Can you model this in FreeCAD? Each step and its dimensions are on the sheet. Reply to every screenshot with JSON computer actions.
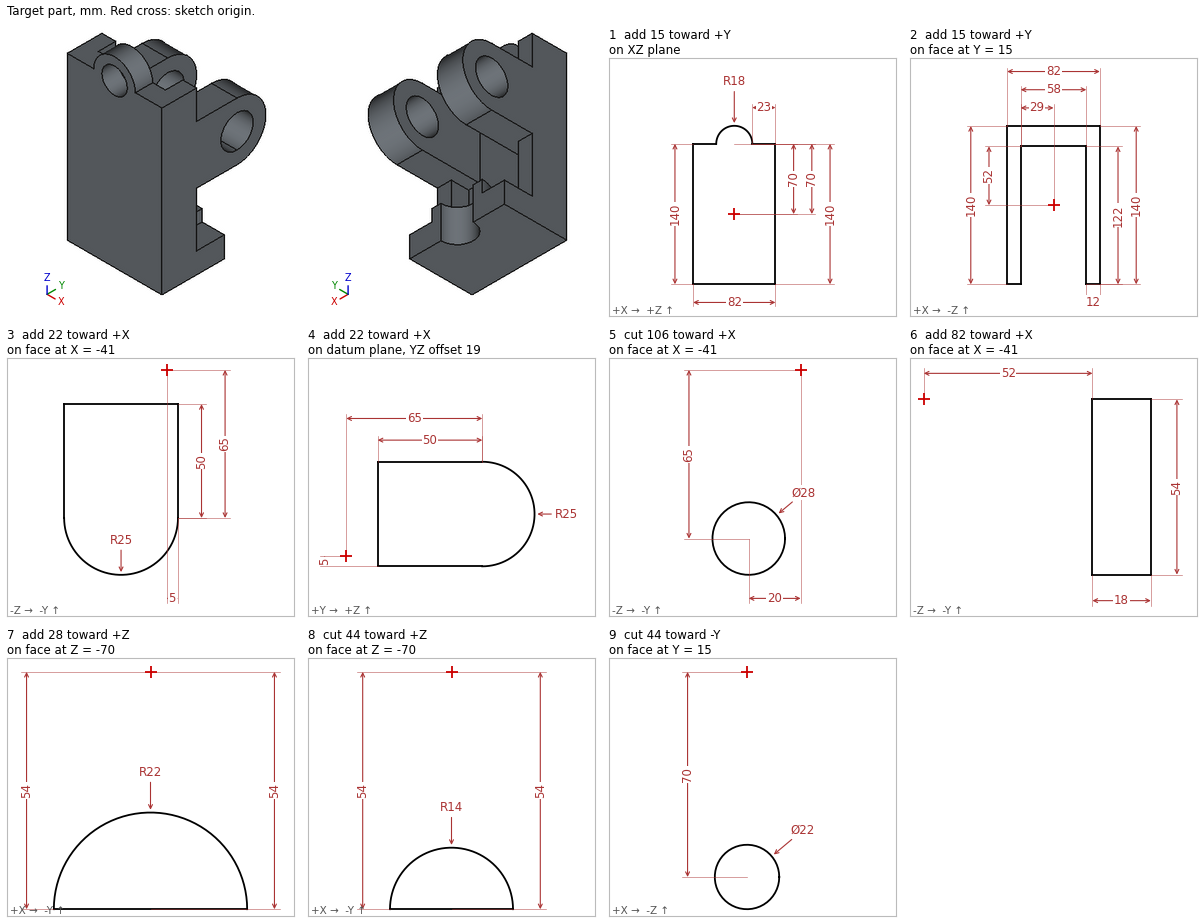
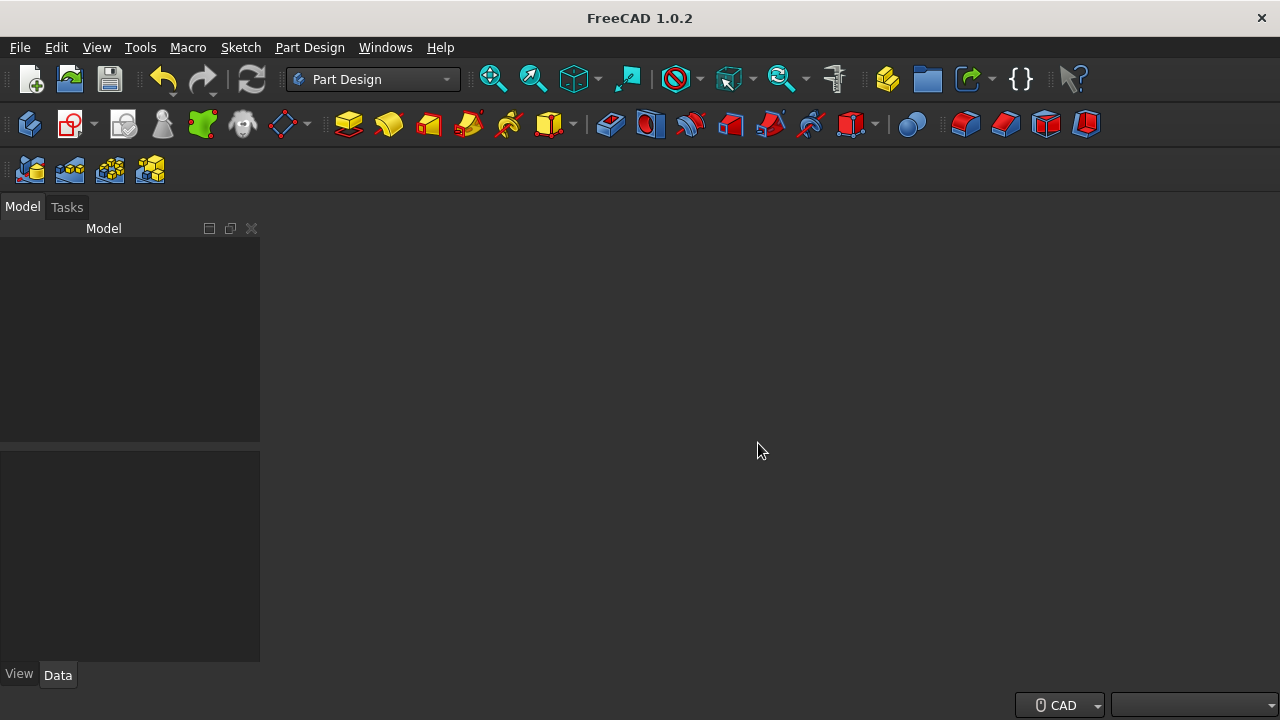
{"action": "left_click", "coordinate": [30, 80]}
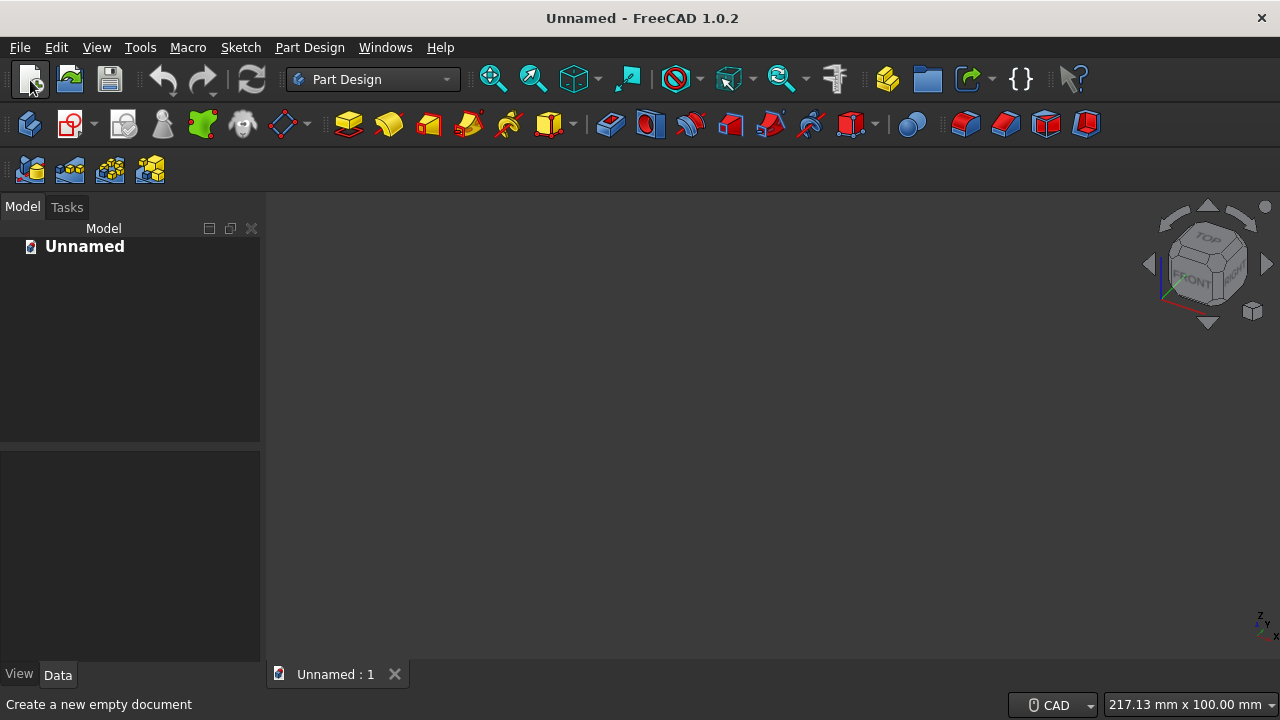
{"action": "left_click", "coordinate": [70, 124]}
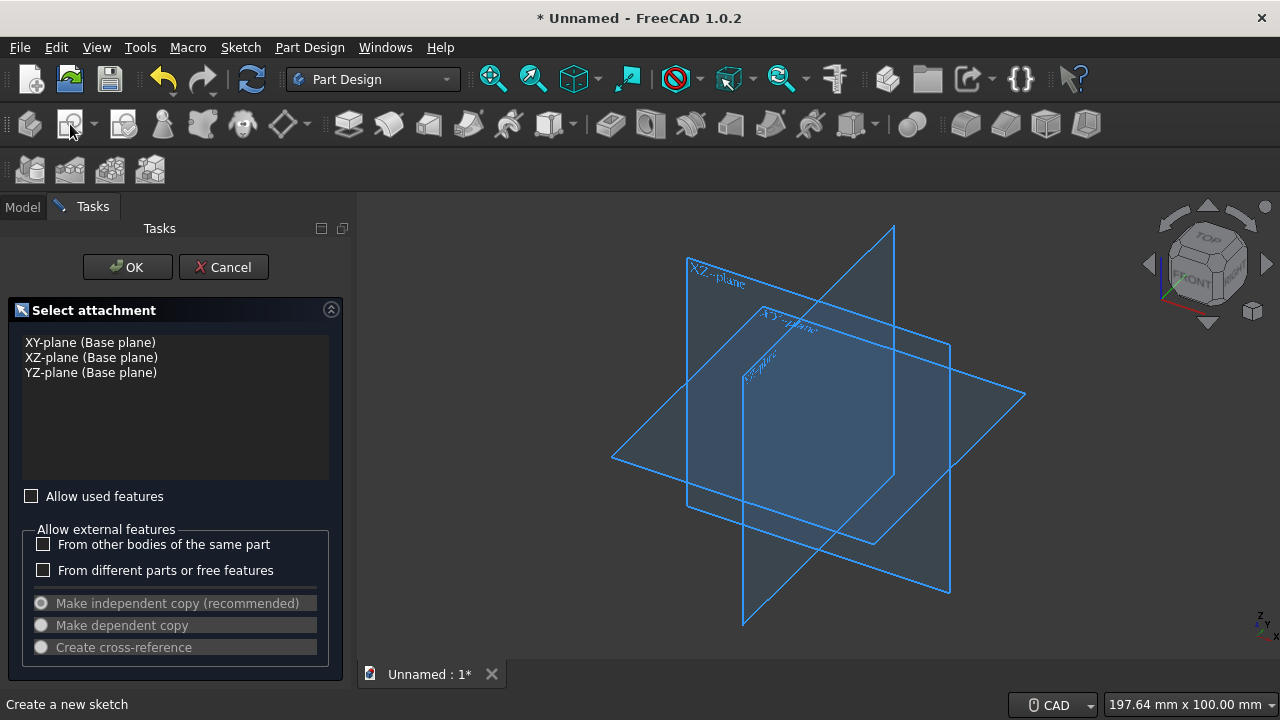
{"action": "left_click", "coordinate": [82, 358]}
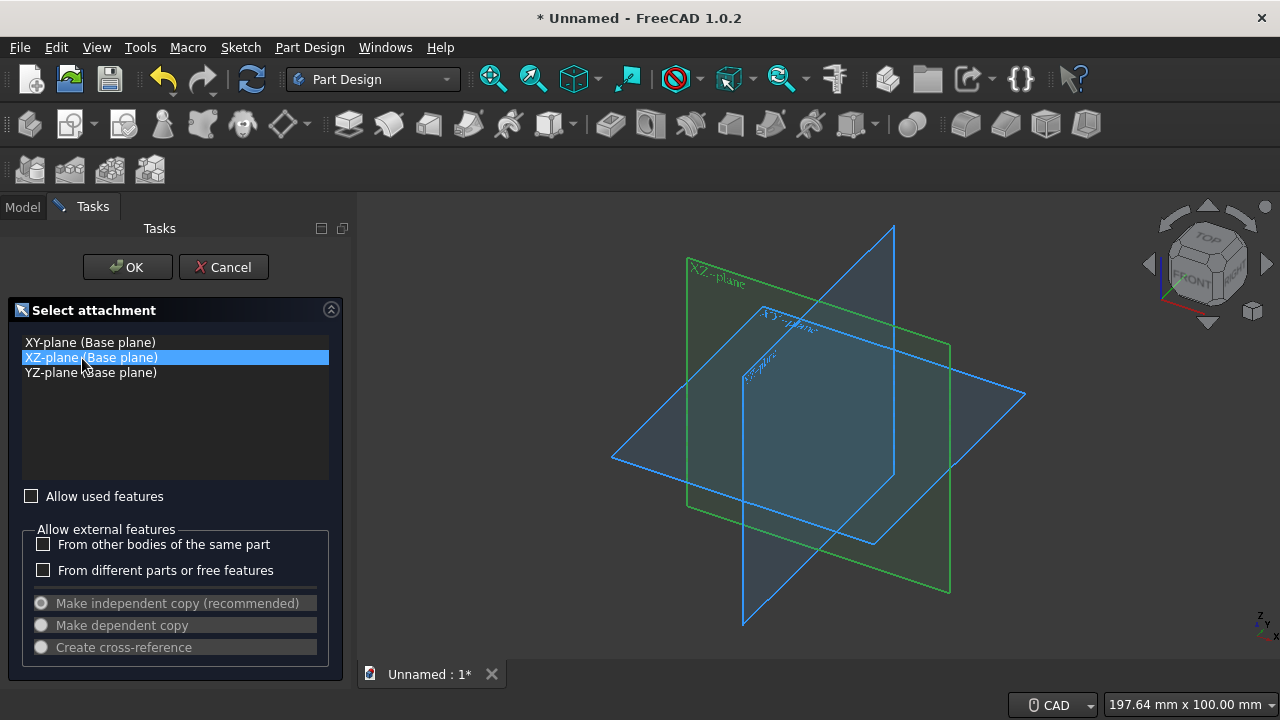
{"action": "left_click", "coordinate": [128, 267]}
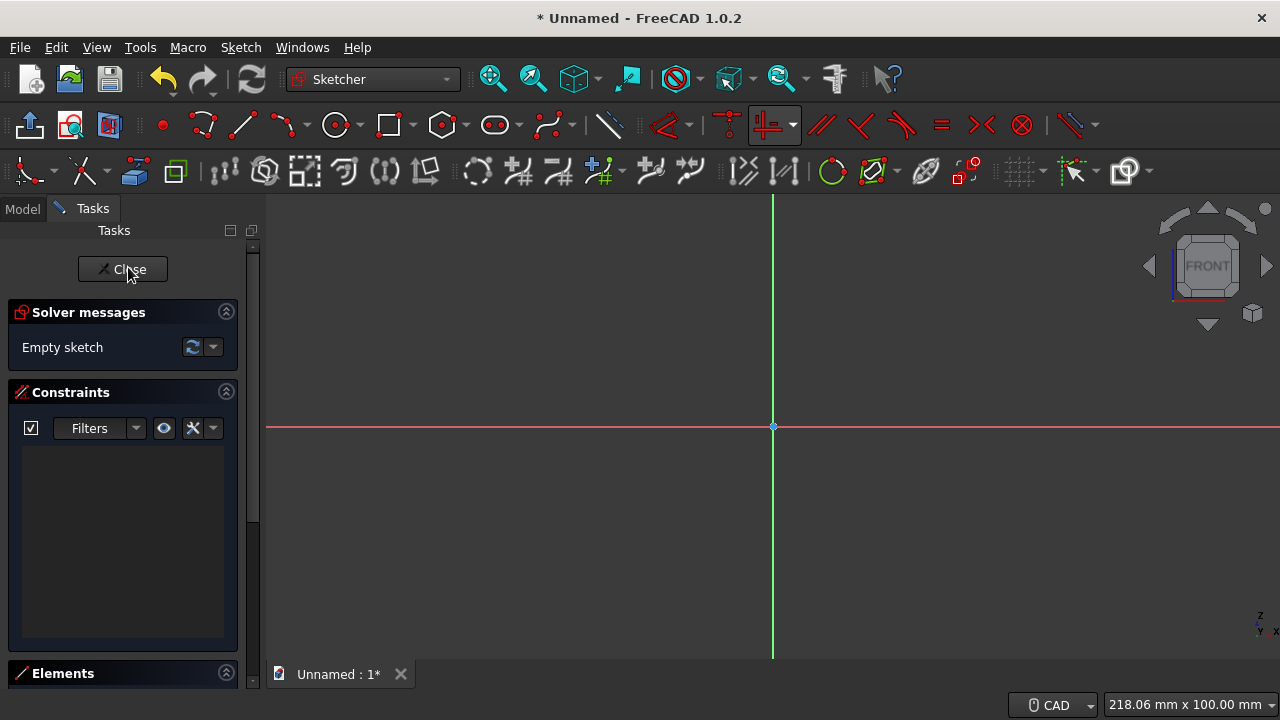
{"action": "scroll", "coordinate": [665, 451], "scroll_direction": "down", "scroll_amount": 5}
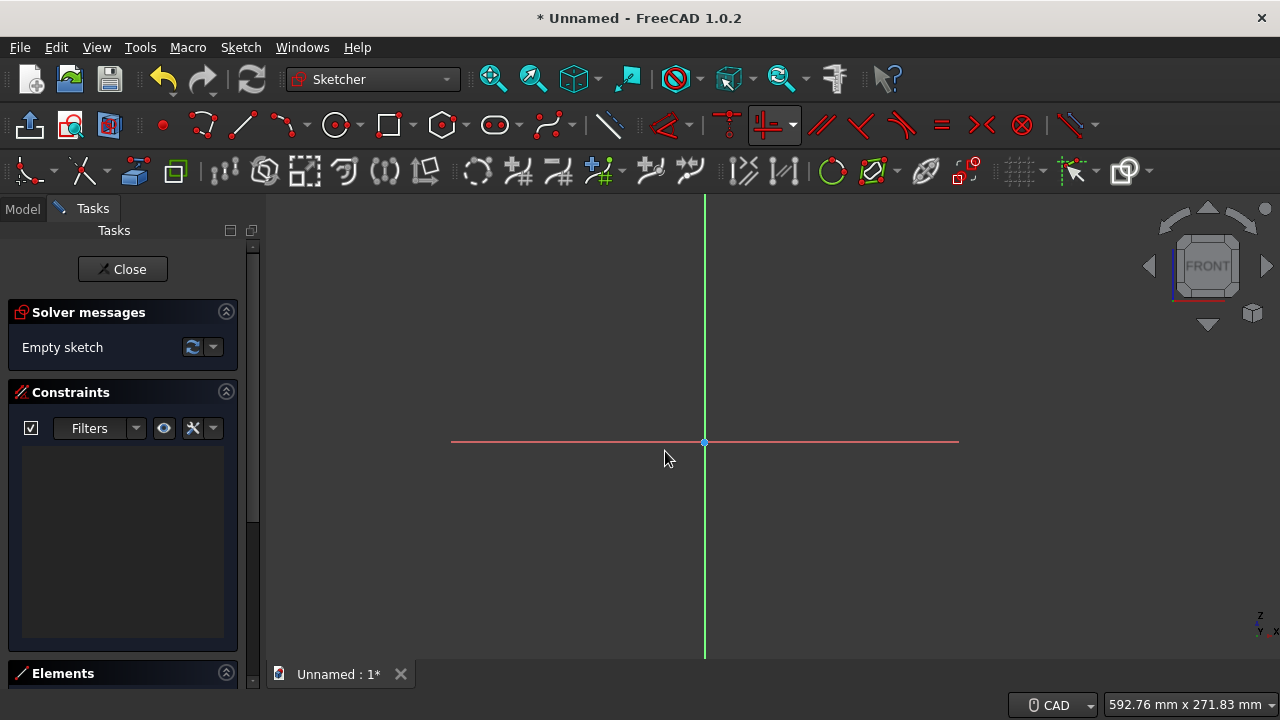
{"action": "left_click", "coordinate": [204, 126]}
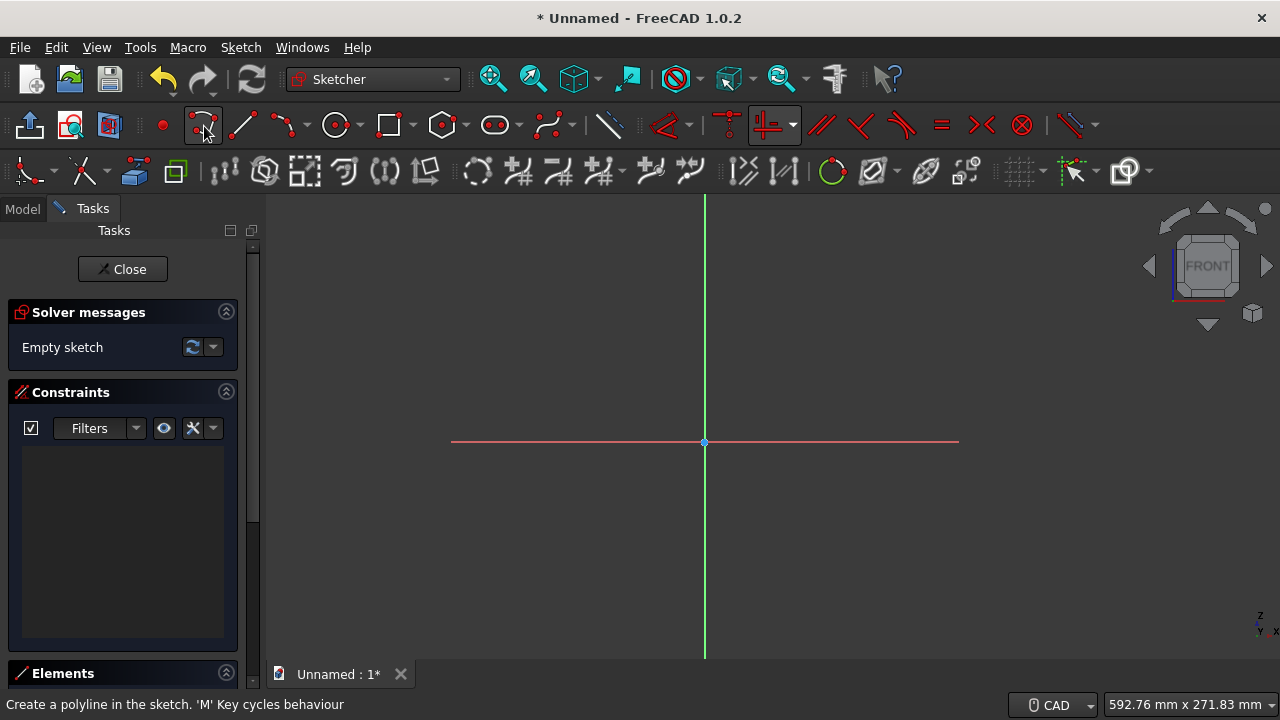
{"action": "left_click", "coordinate": [736, 323]}
{"action": "left_click", "coordinate": [775, 323]}
{"action": "left_click", "coordinate": [775, 562]}
{"action": "left_click", "coordinate": [635, 562]}
{"action": "left_click", "coordinate": [635, 323]}
{"action": "left_click", "coordinate": [674, 323]}
{"action": "right_click", "coordinate": [674, 323]}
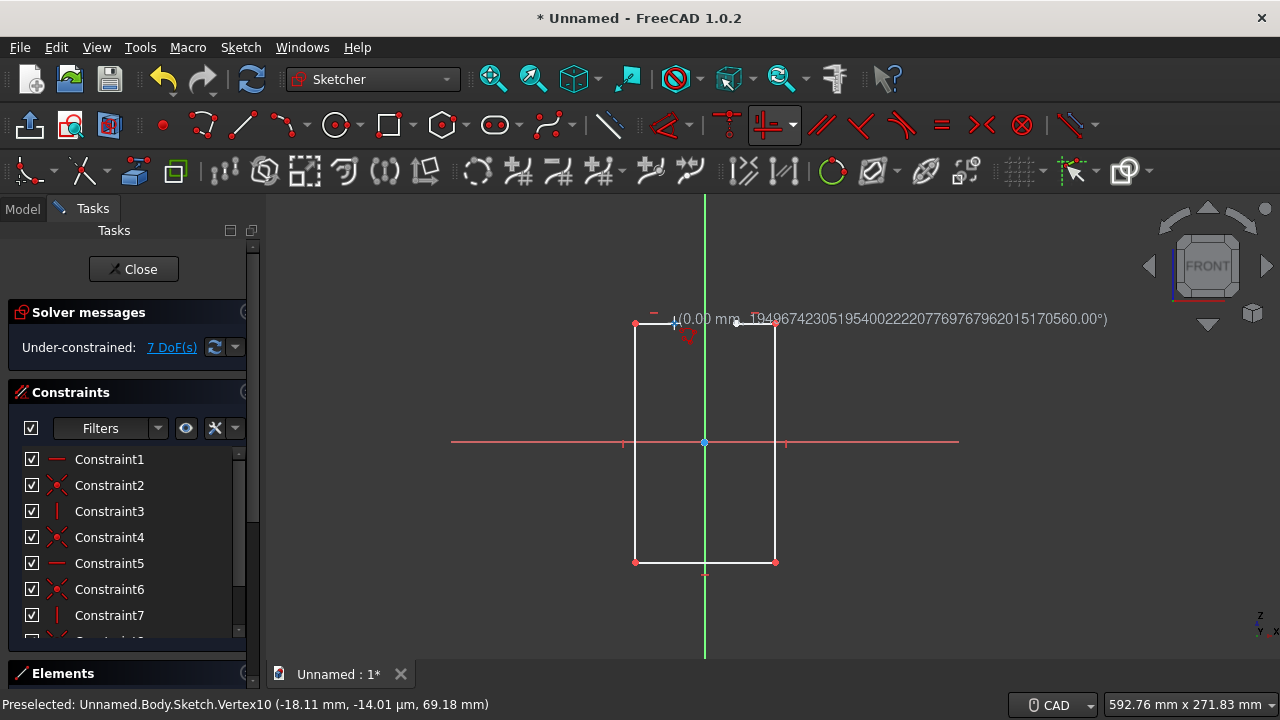
{"action": "key", "text": "g 3 a"}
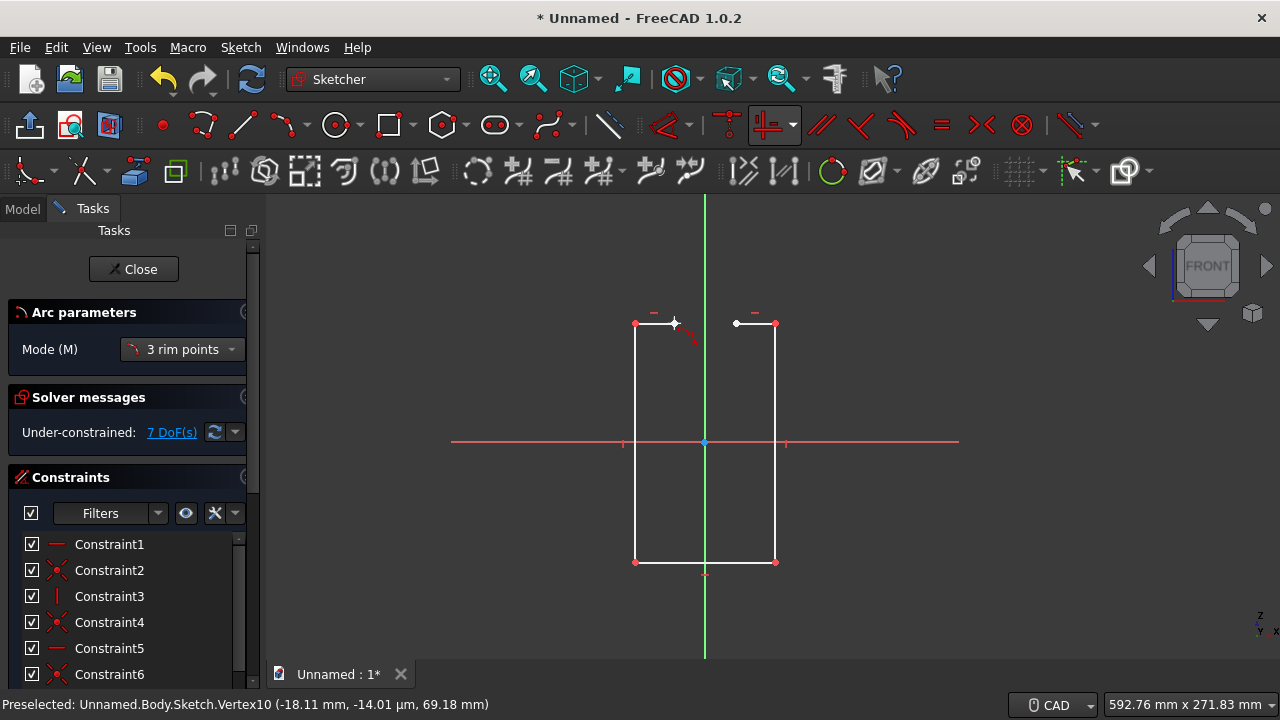
{"action": "left_click", "coordinate": [674, 324]}
{"action": "left_click", "coordinate": [736, 324]}
{"action": "left_click", "coordinate": [723, 298]}
{"action": "key", "text": "Escape"}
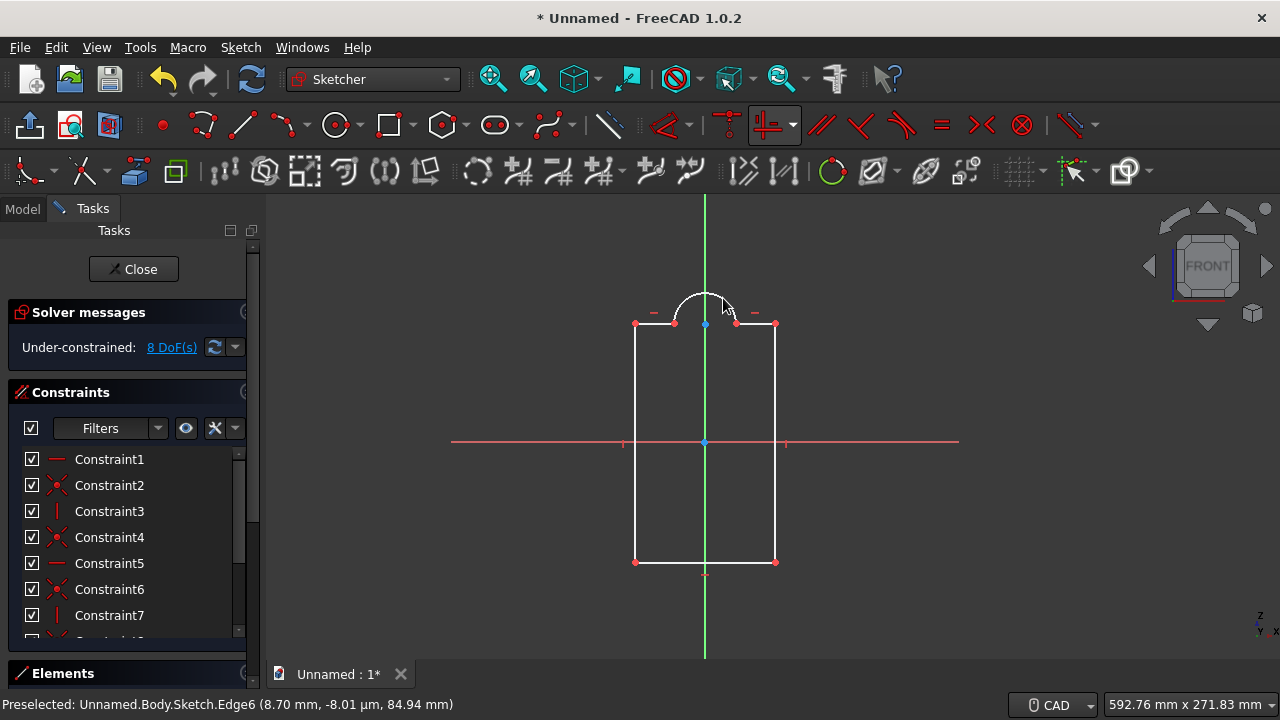
{"action": "left_click", "coordinate": [705, 324]}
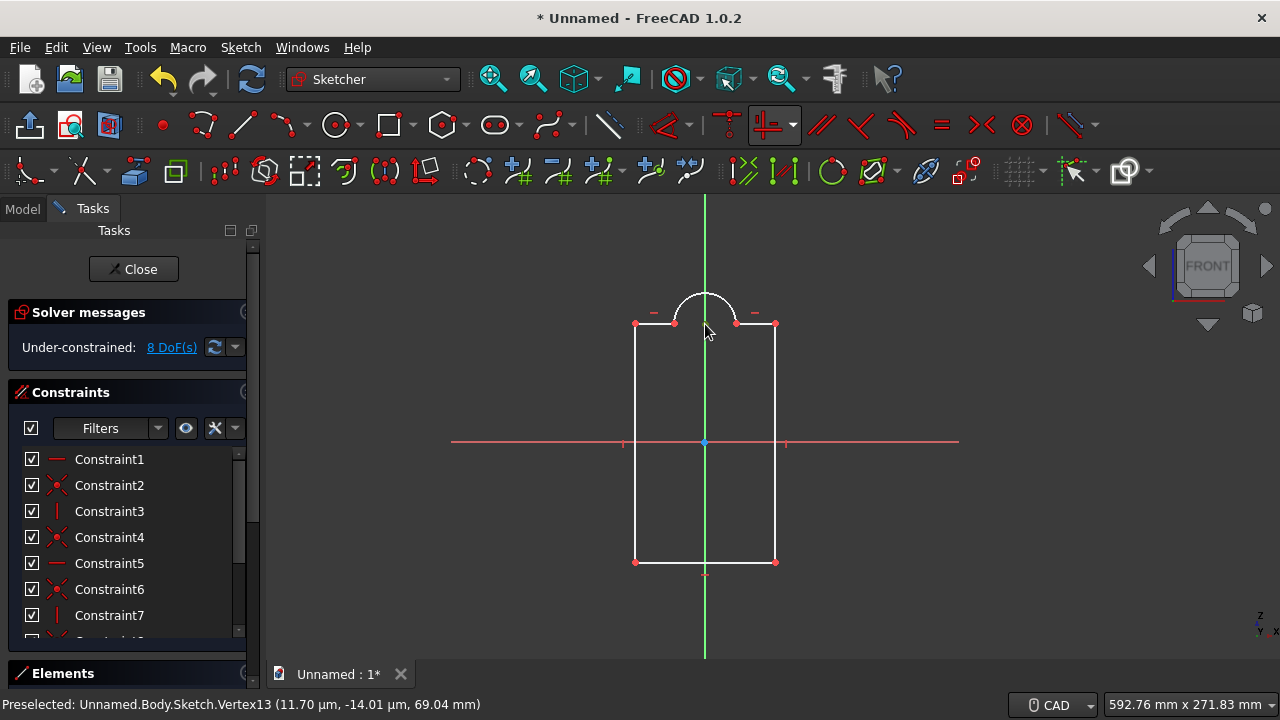
{"action": "left_click", "coordinate": [705, 602]}